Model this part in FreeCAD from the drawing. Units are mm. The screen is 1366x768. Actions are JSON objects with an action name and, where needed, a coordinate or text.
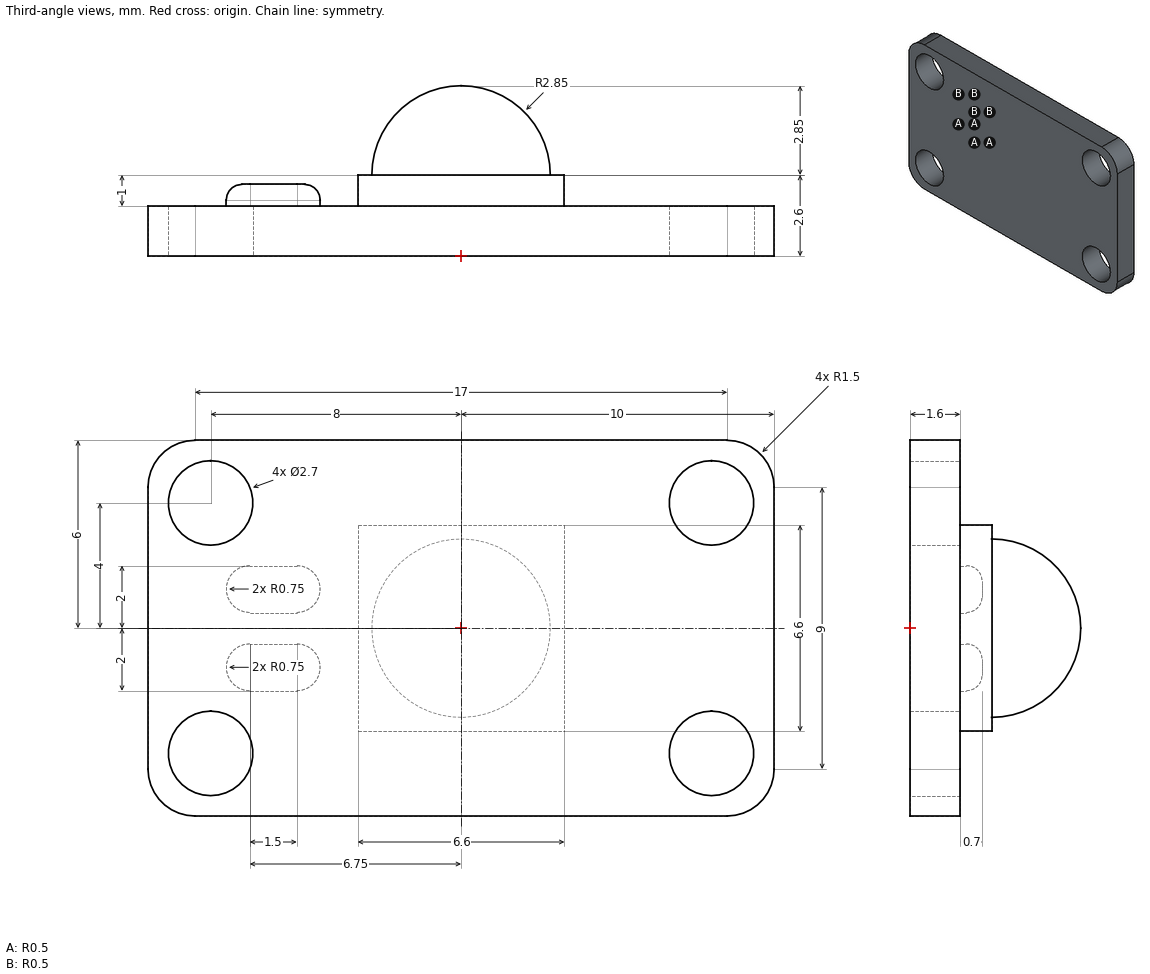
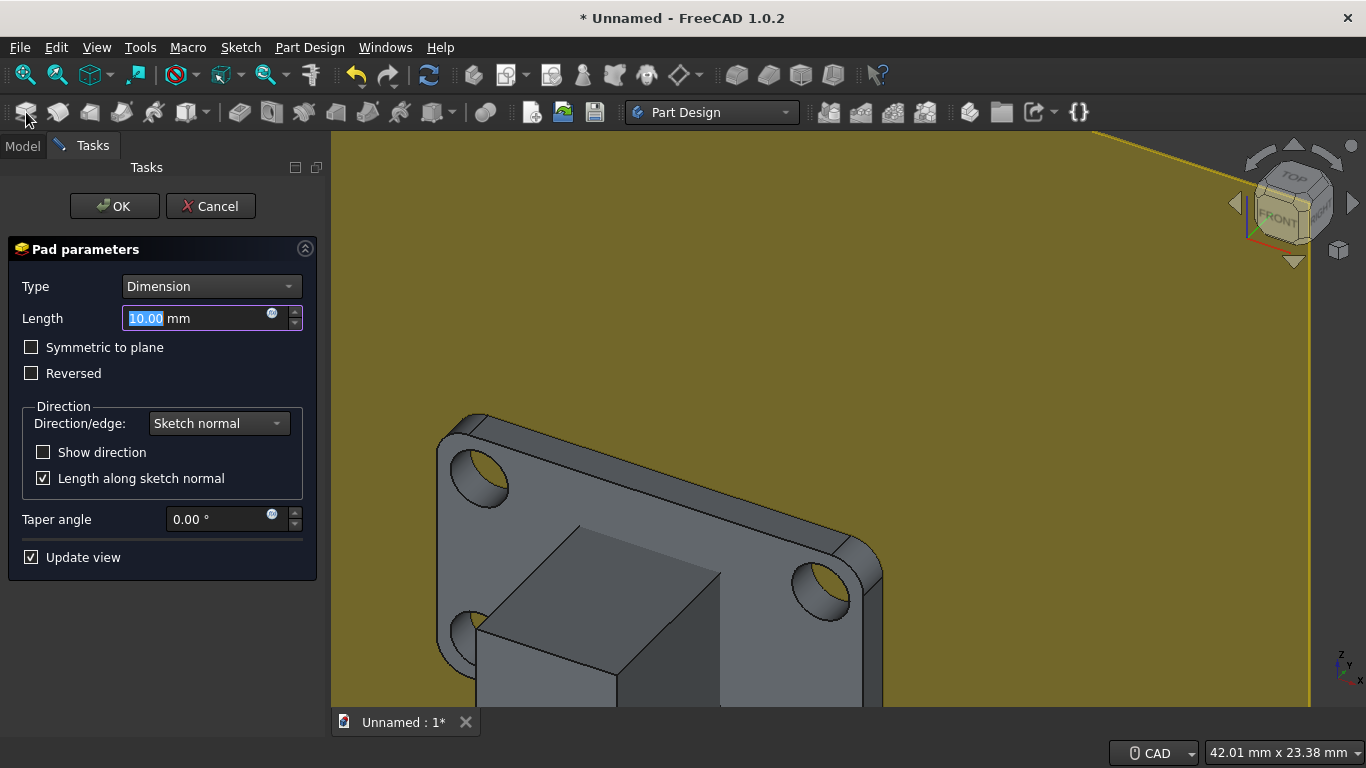
{"action": "type", "text": "1"}
{"action": "key", "text": "Tab"}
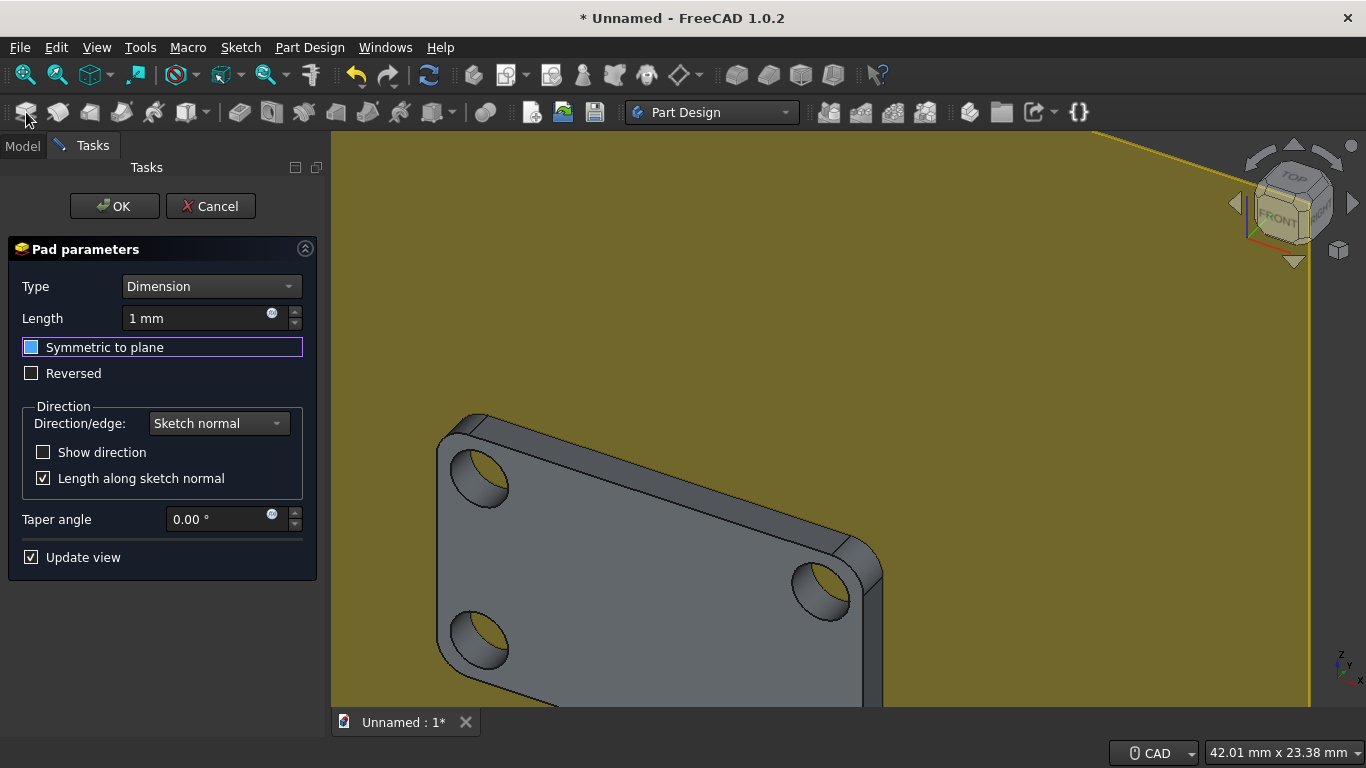
{"action": "left_click", "coordinate": [30, 373]}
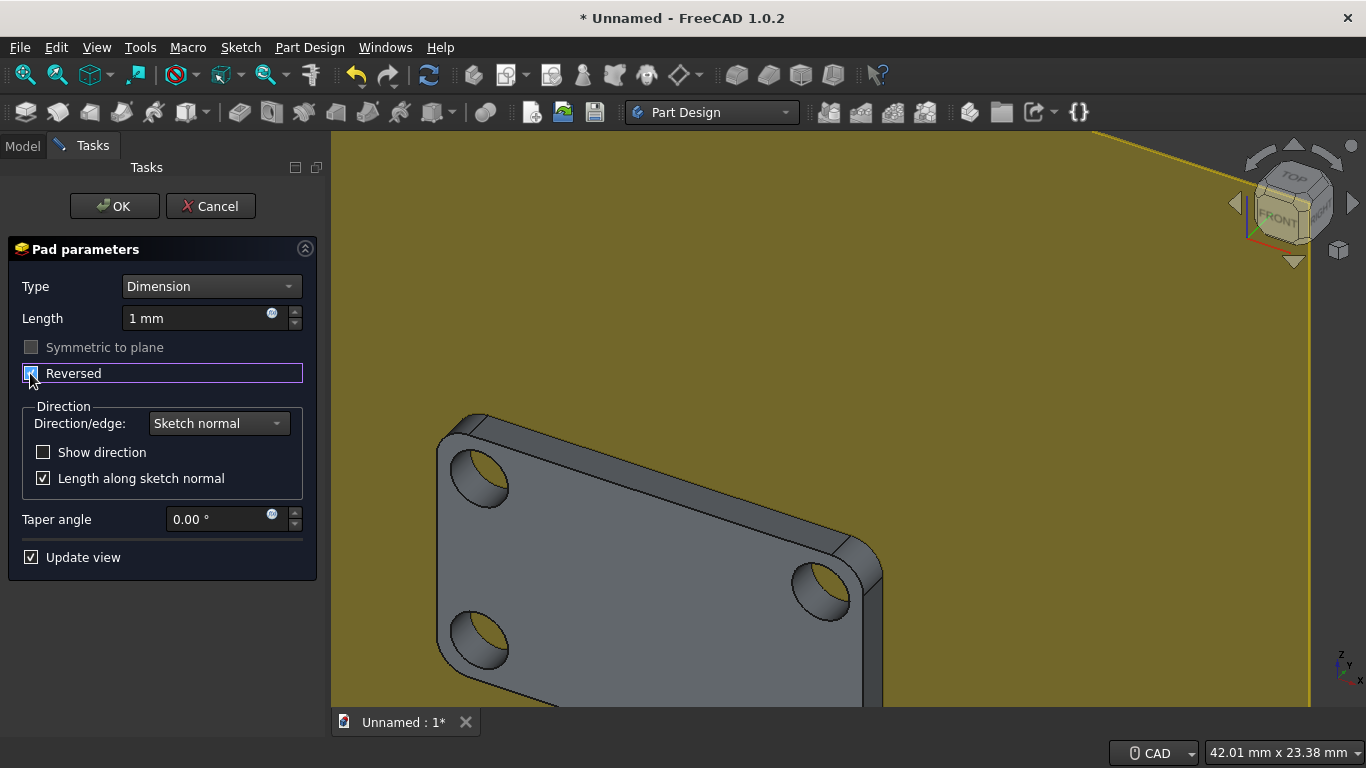
{"action": "left_click", "coordinate": [115, 206]}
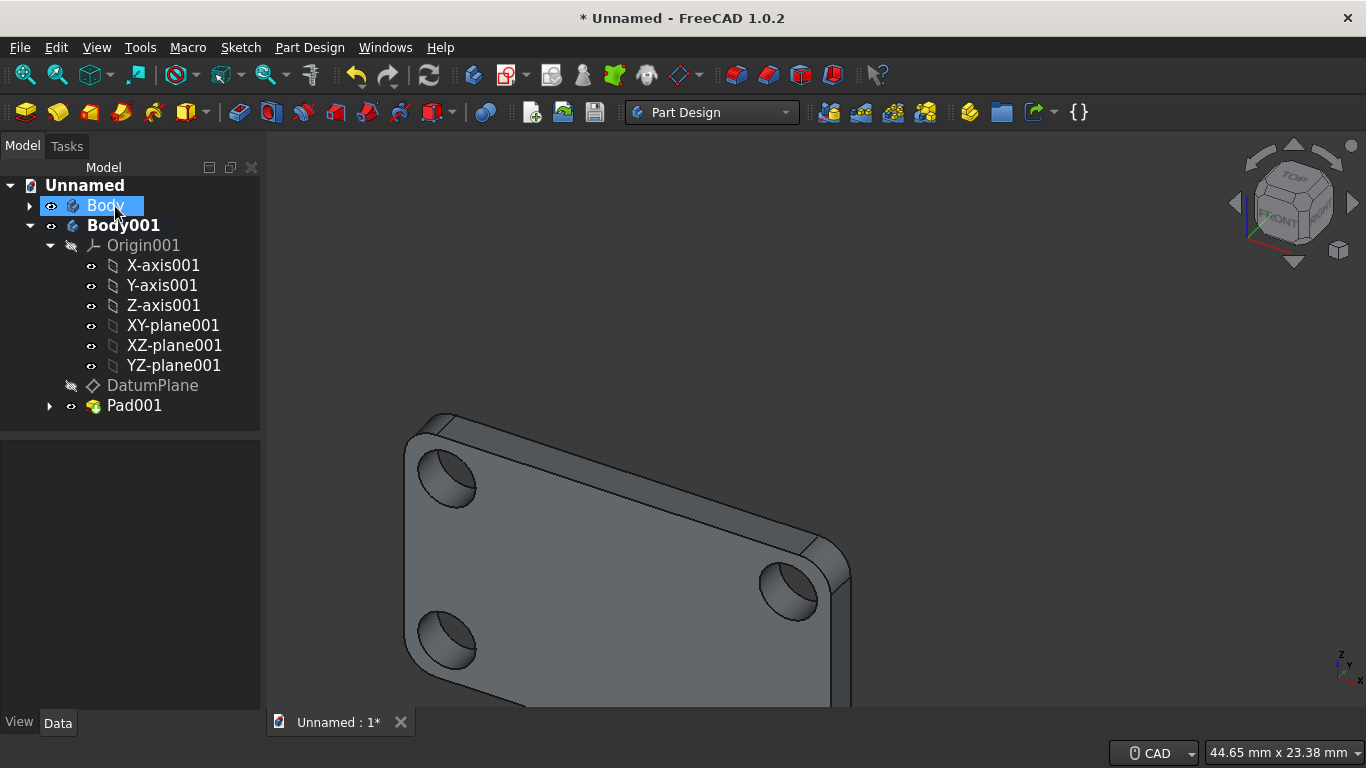
{"action": "left_click", "coordinate": [26, 76]}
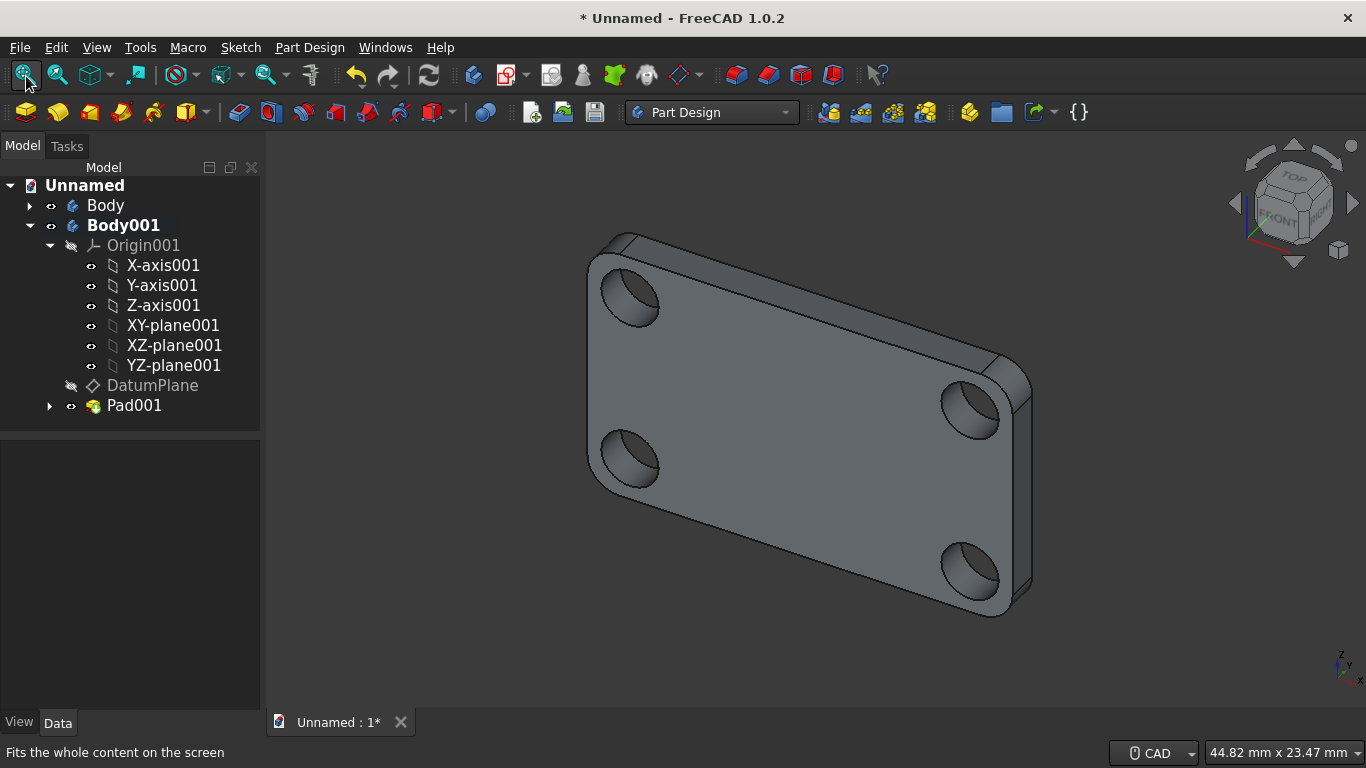
{"action": "left_click", "coordinate": [506, 76]}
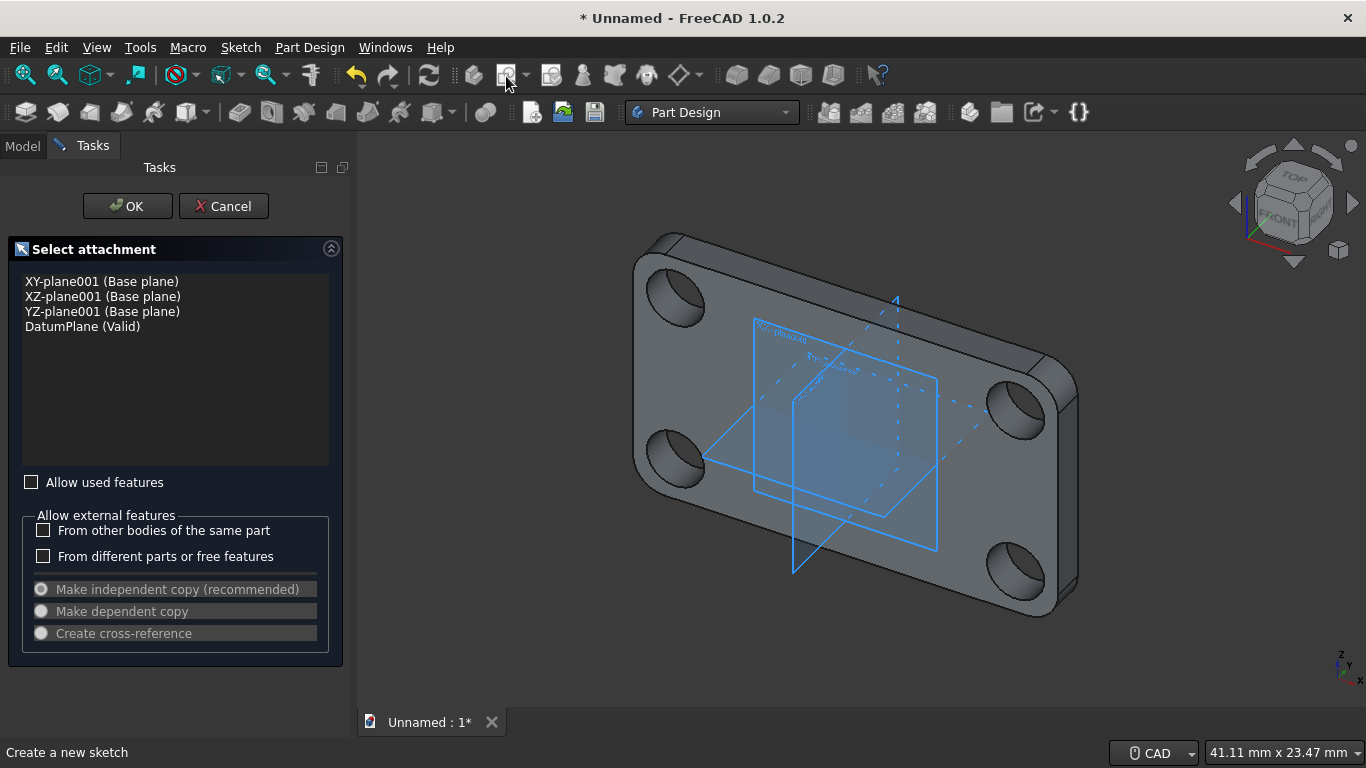
{"action": "left_click", "coordinate": [82, 282]}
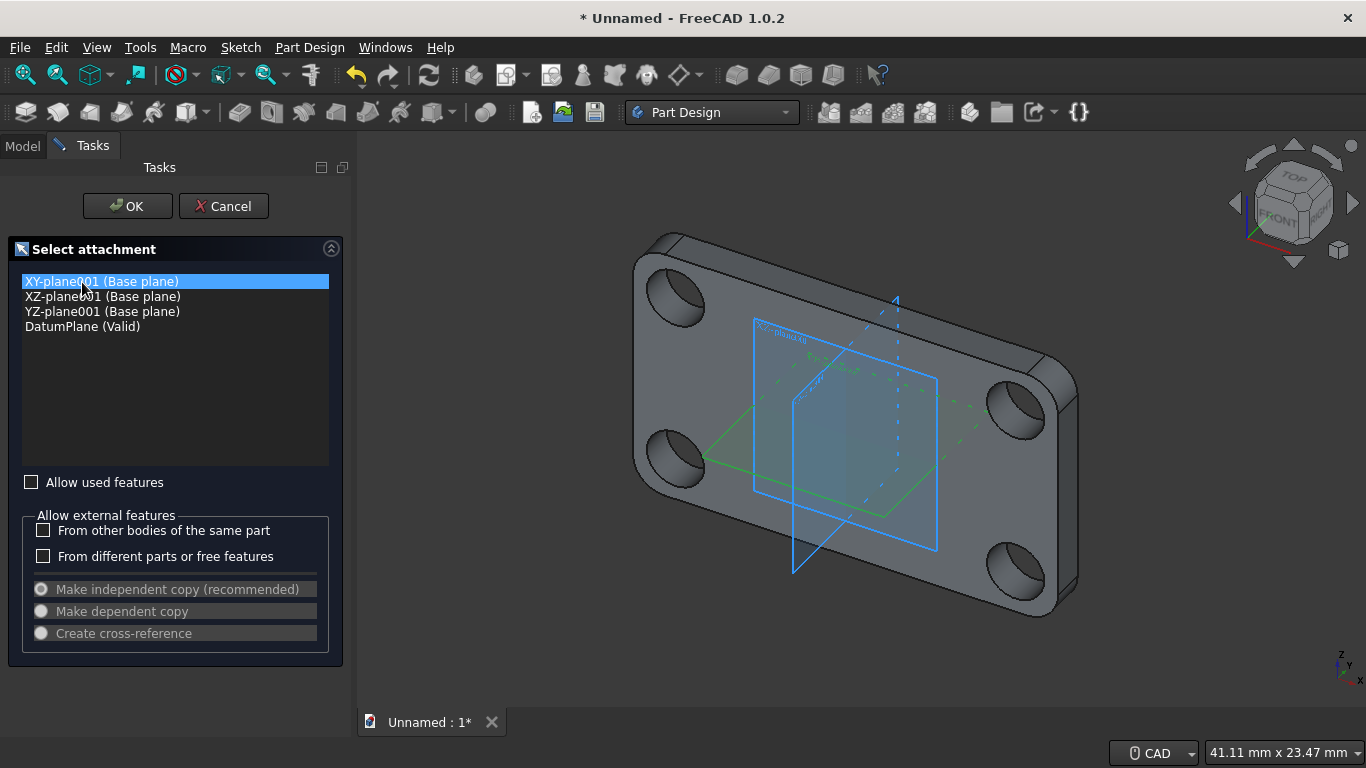
{"action": "left_click", "coordinate": [128, 206]}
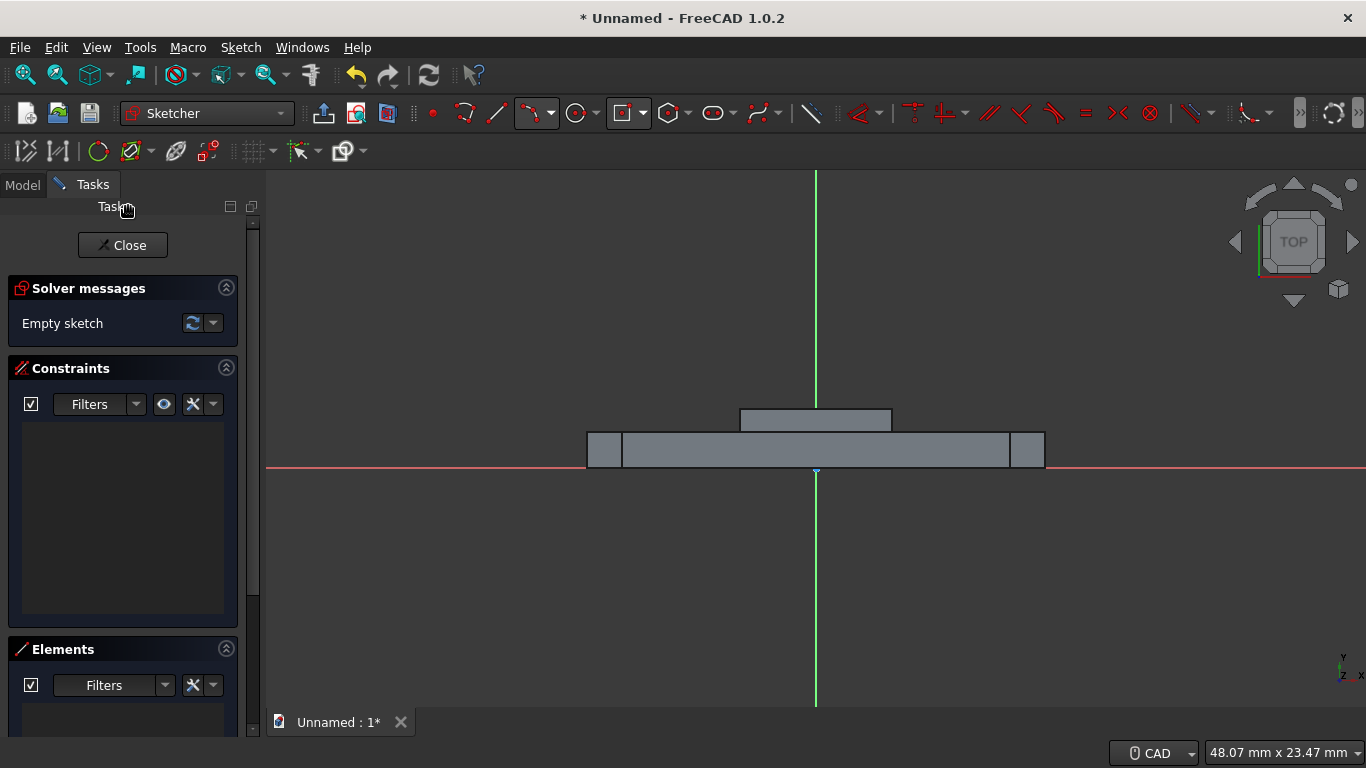
{"action": "left_click", "coordinate": [388, 114]}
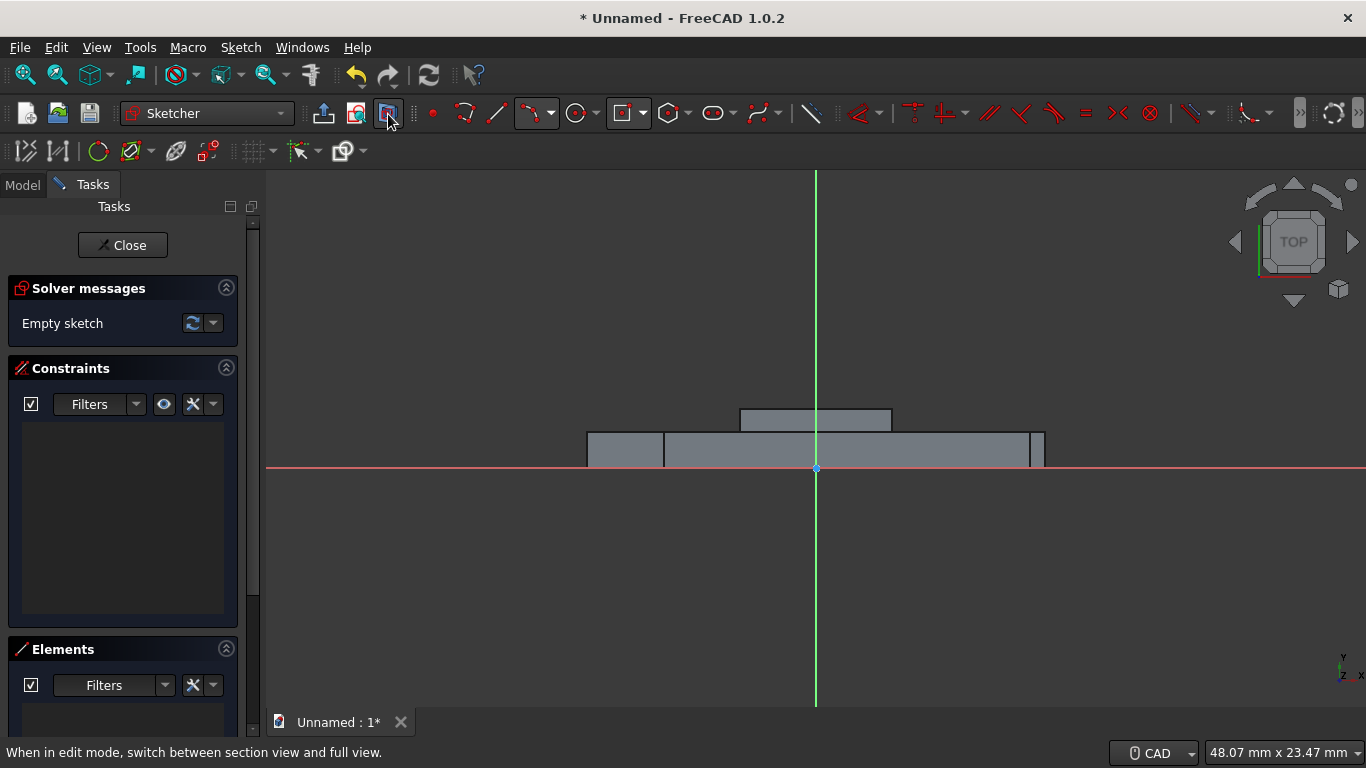
{"action": "scroll", "coordinate": [907, 387], "scroll_direction": "up", "scroll_amount": 5}